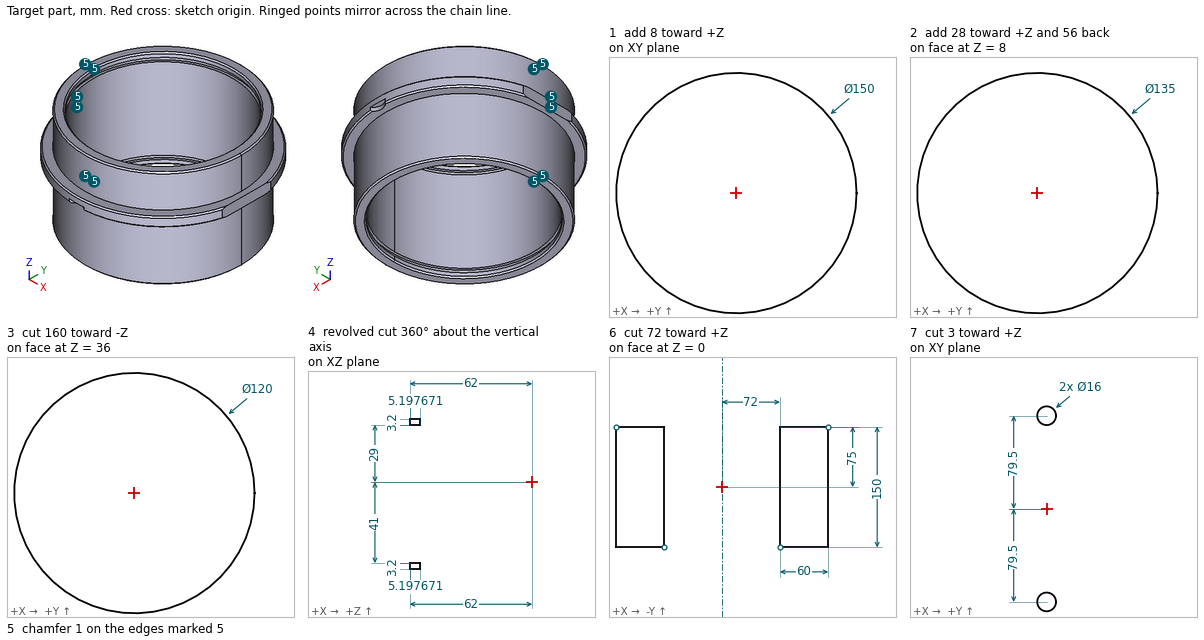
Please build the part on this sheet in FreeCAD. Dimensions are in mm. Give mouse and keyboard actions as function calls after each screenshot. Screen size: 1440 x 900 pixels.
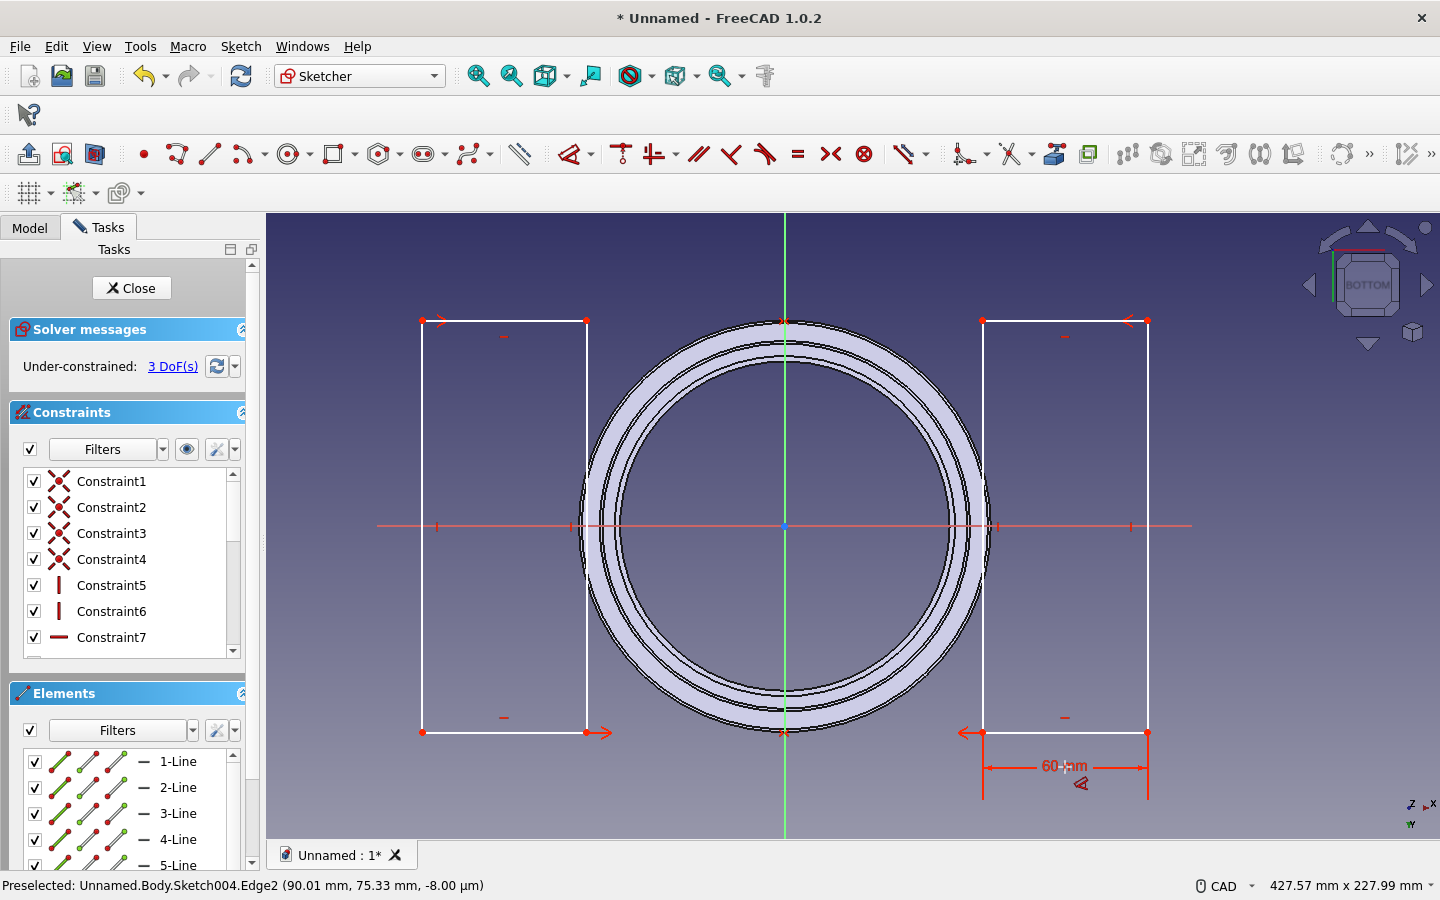
click(983, 445)
click(1017, 432)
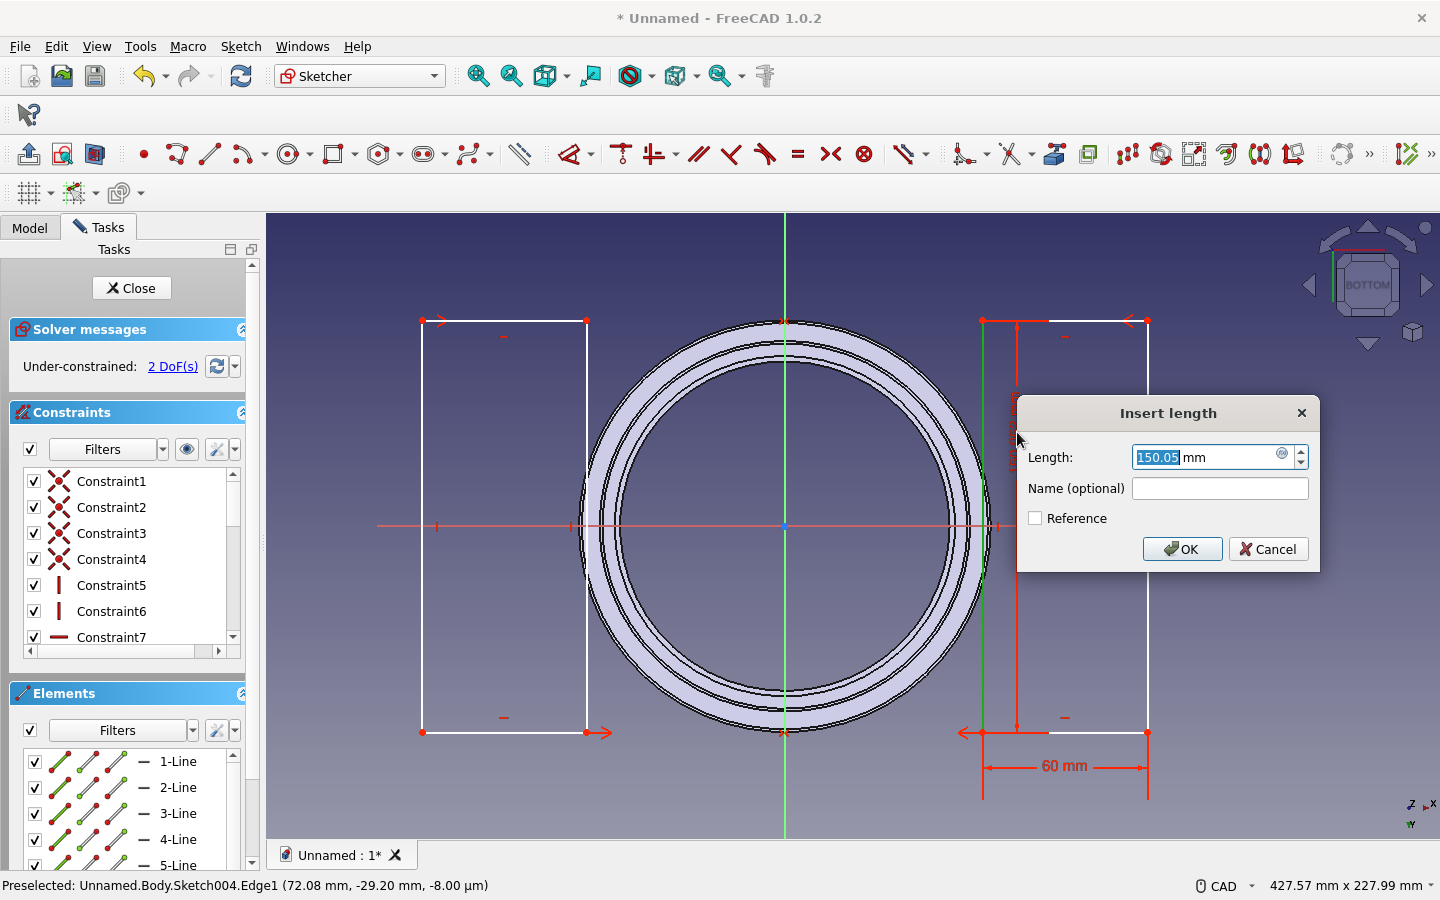
text(150)
key(Return)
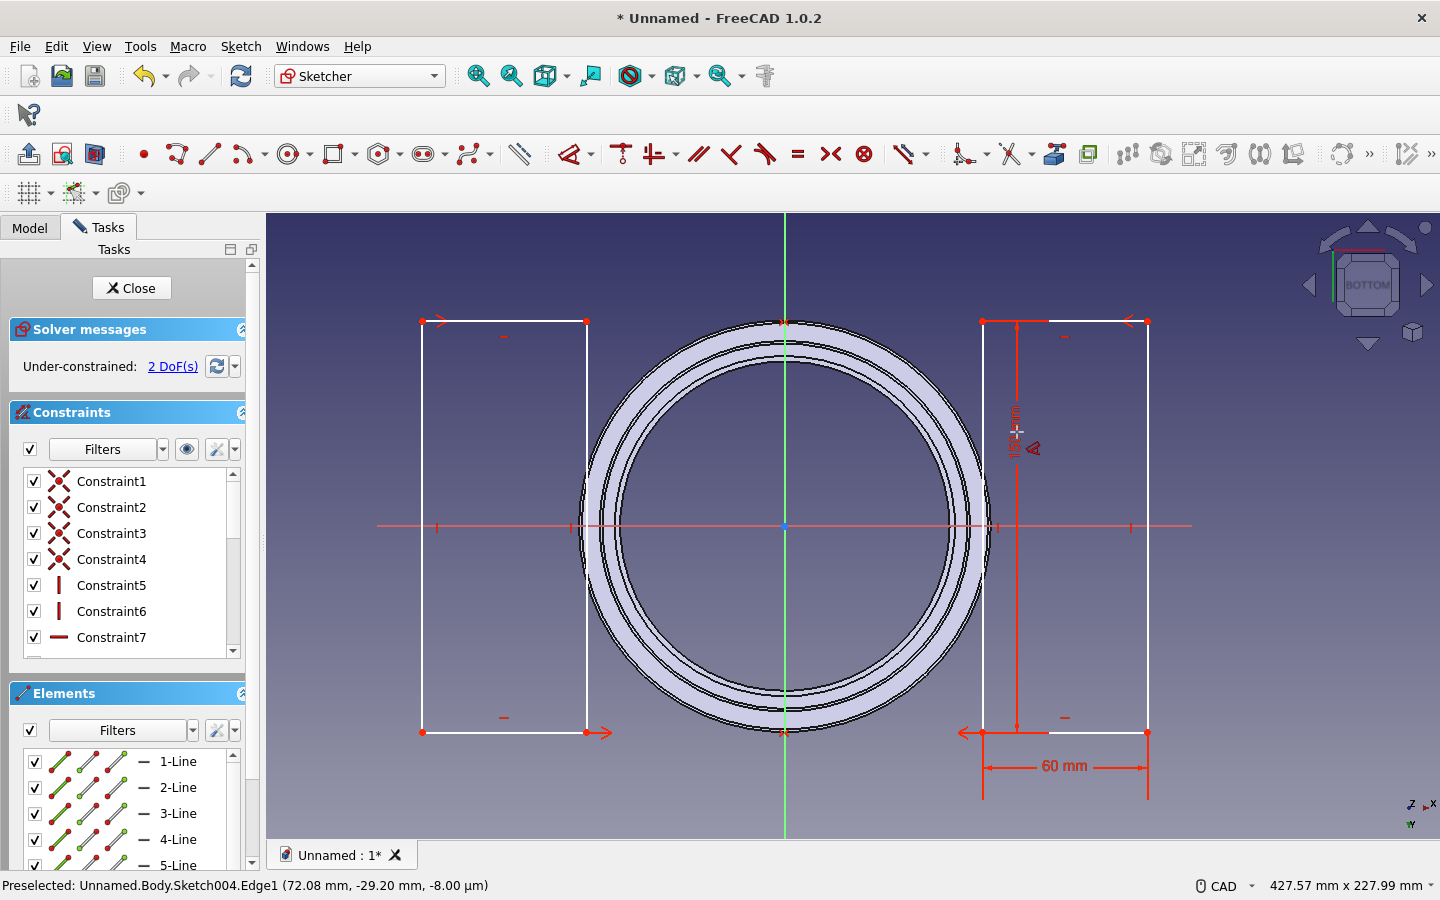
click(983, 321)
click(884, 287)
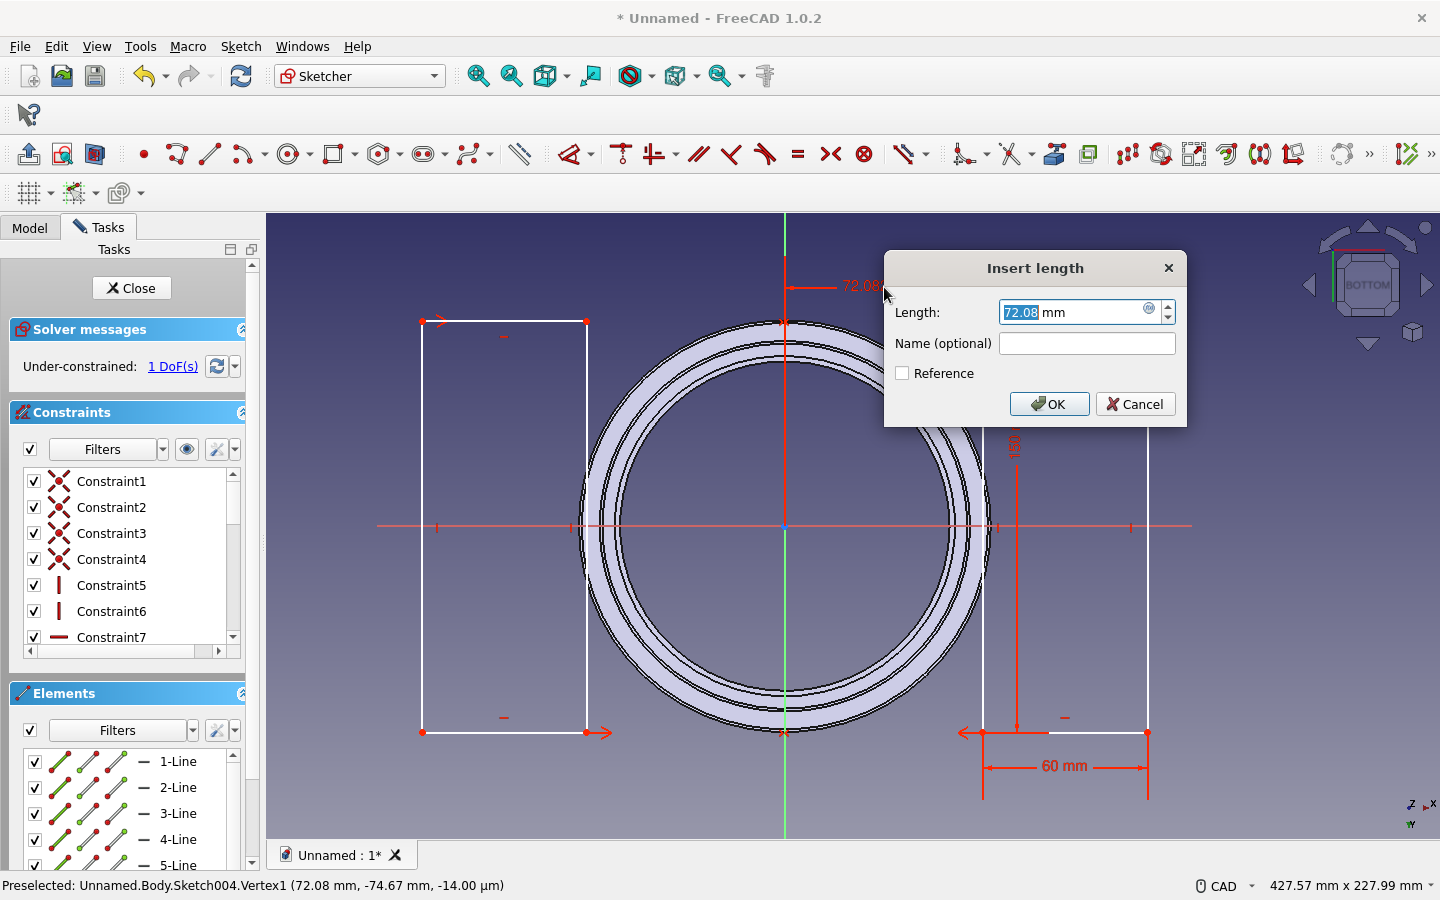
text(72)
key(Return)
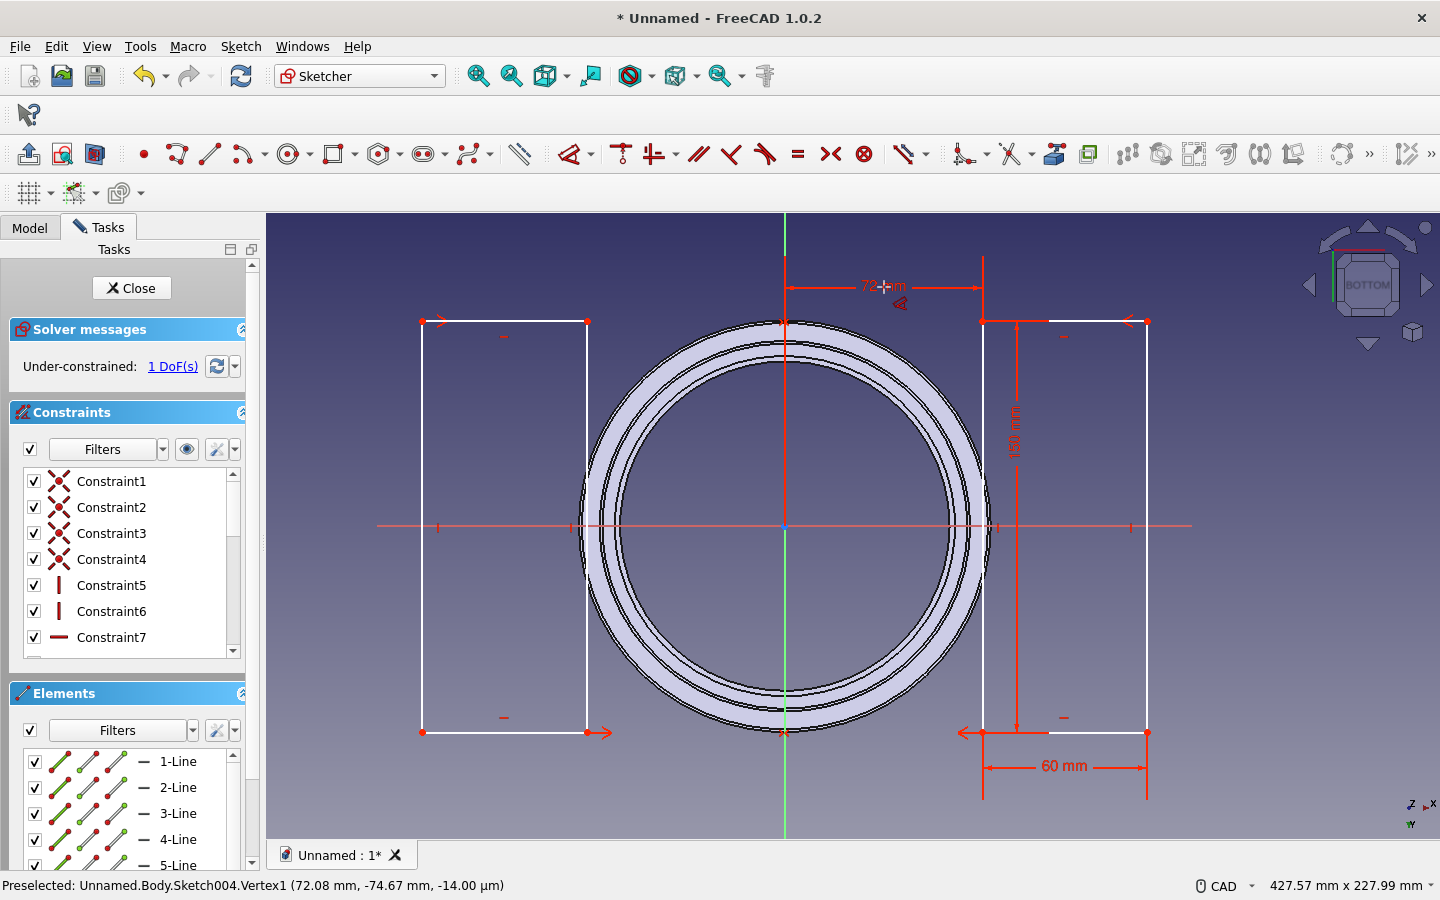
click(983, 321)
click(1017, 376)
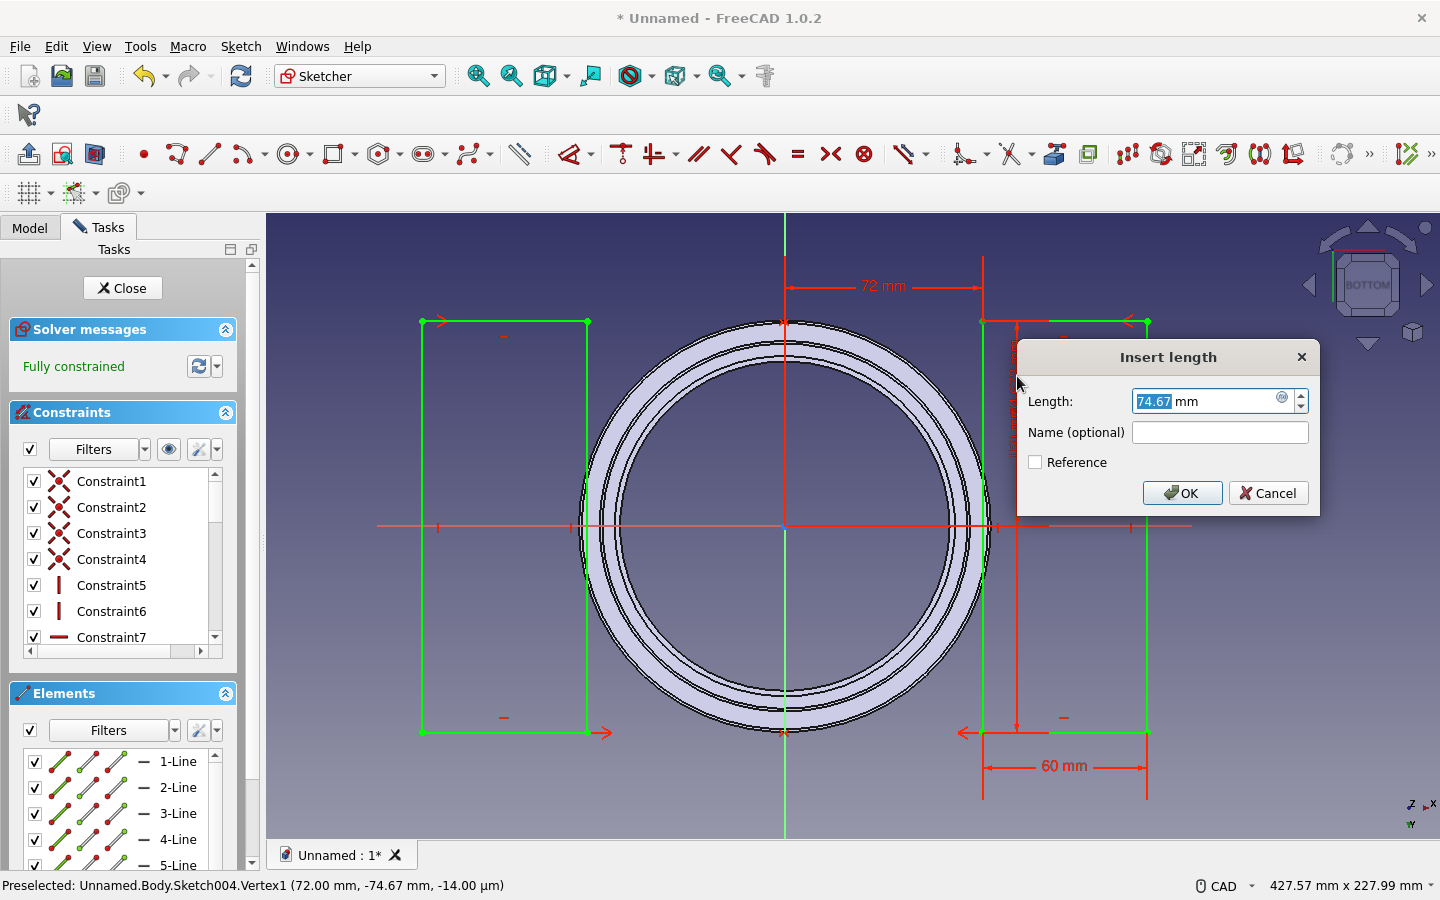
text(75)
key(Return)
key(Escape)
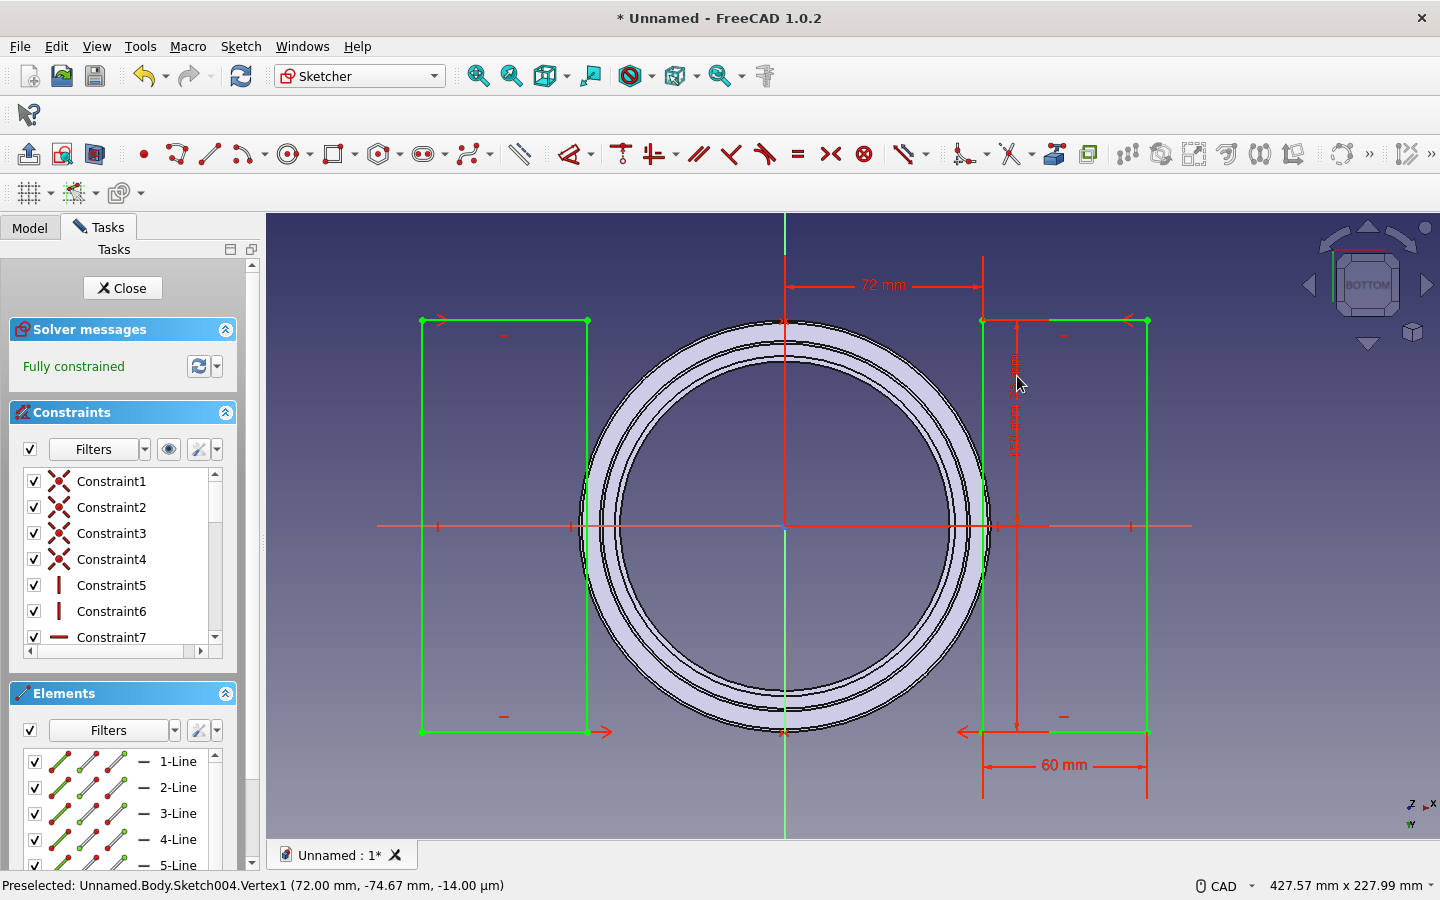
click(123, 288)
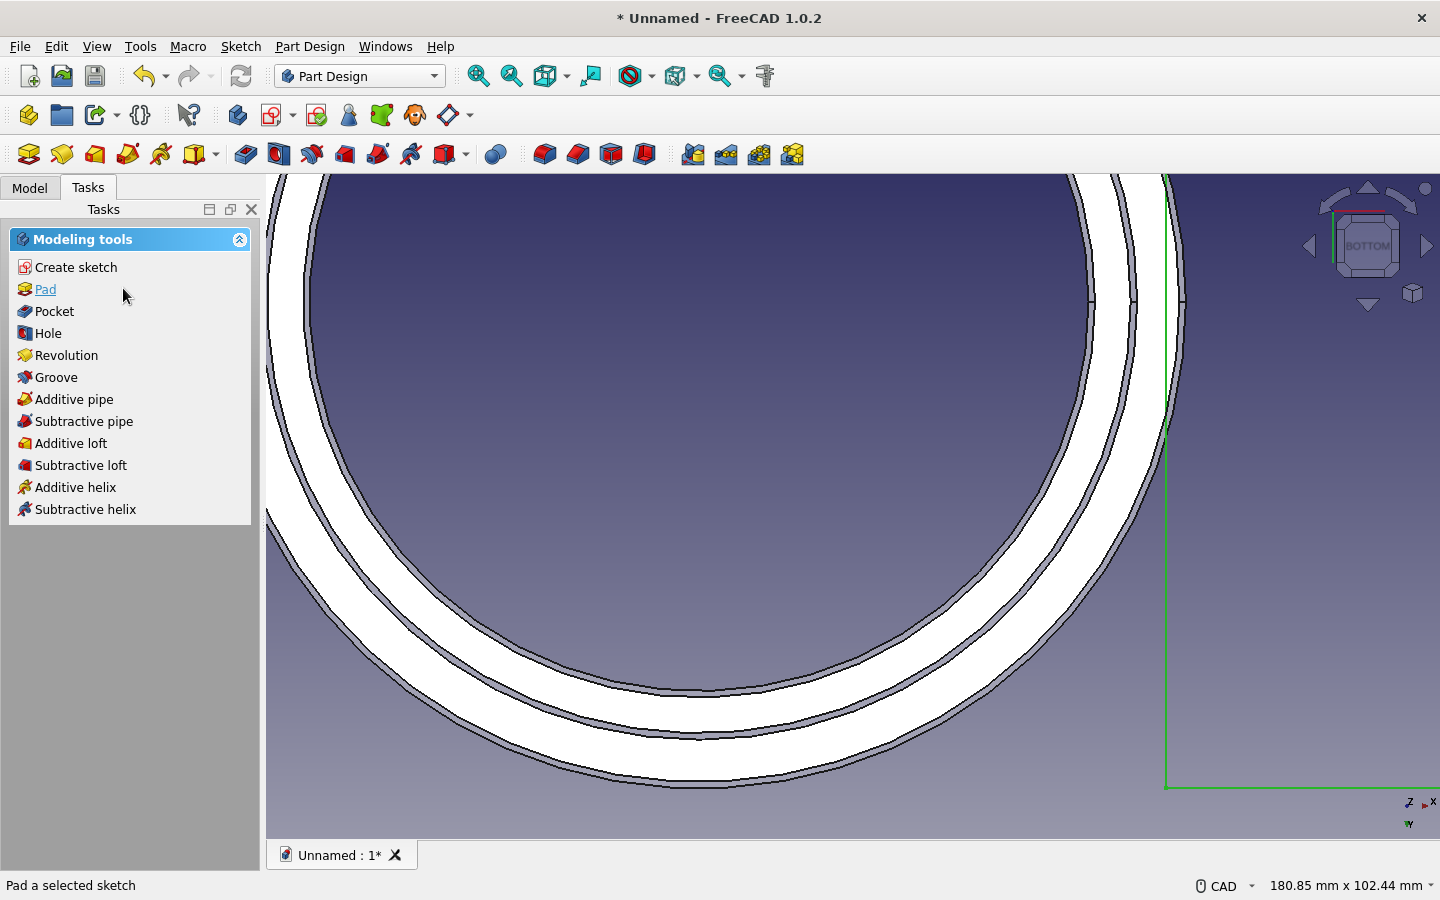
click(246, 154)